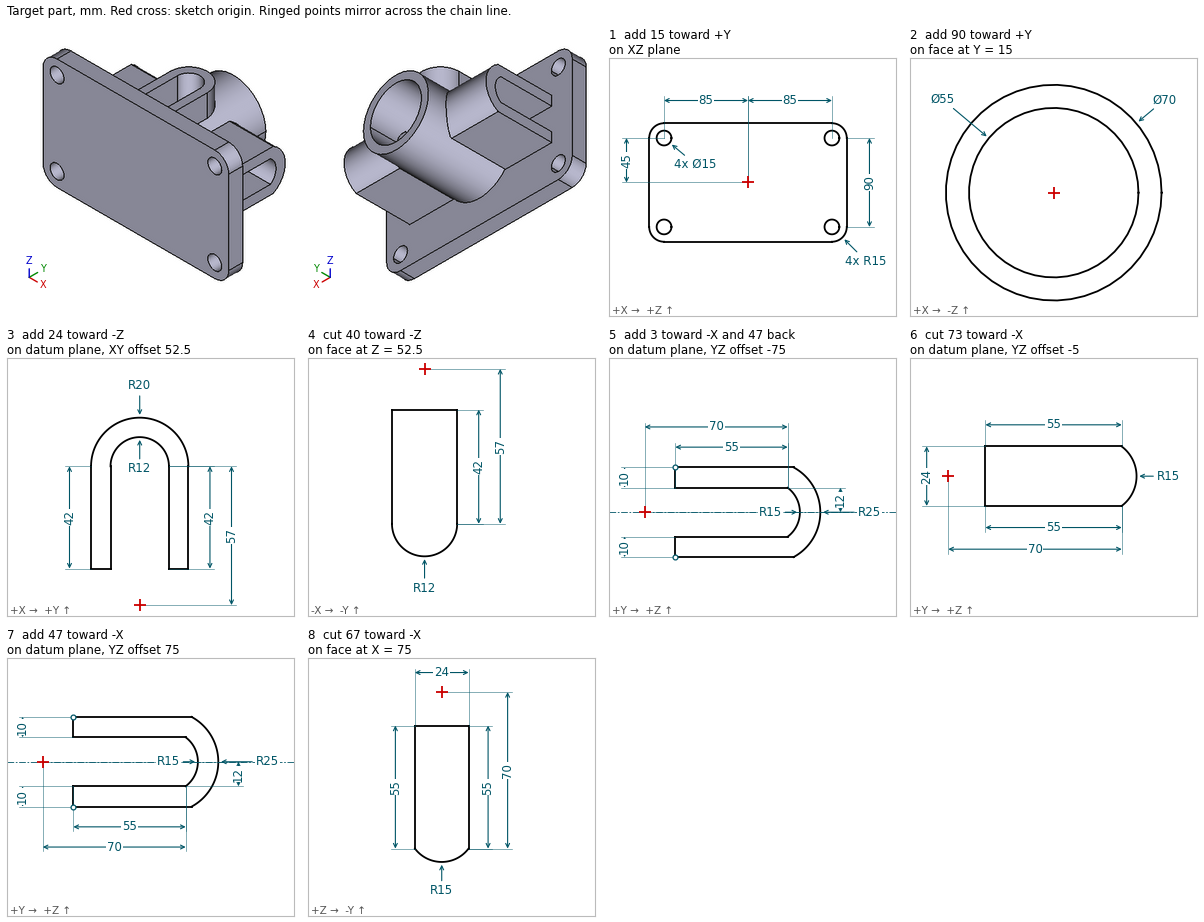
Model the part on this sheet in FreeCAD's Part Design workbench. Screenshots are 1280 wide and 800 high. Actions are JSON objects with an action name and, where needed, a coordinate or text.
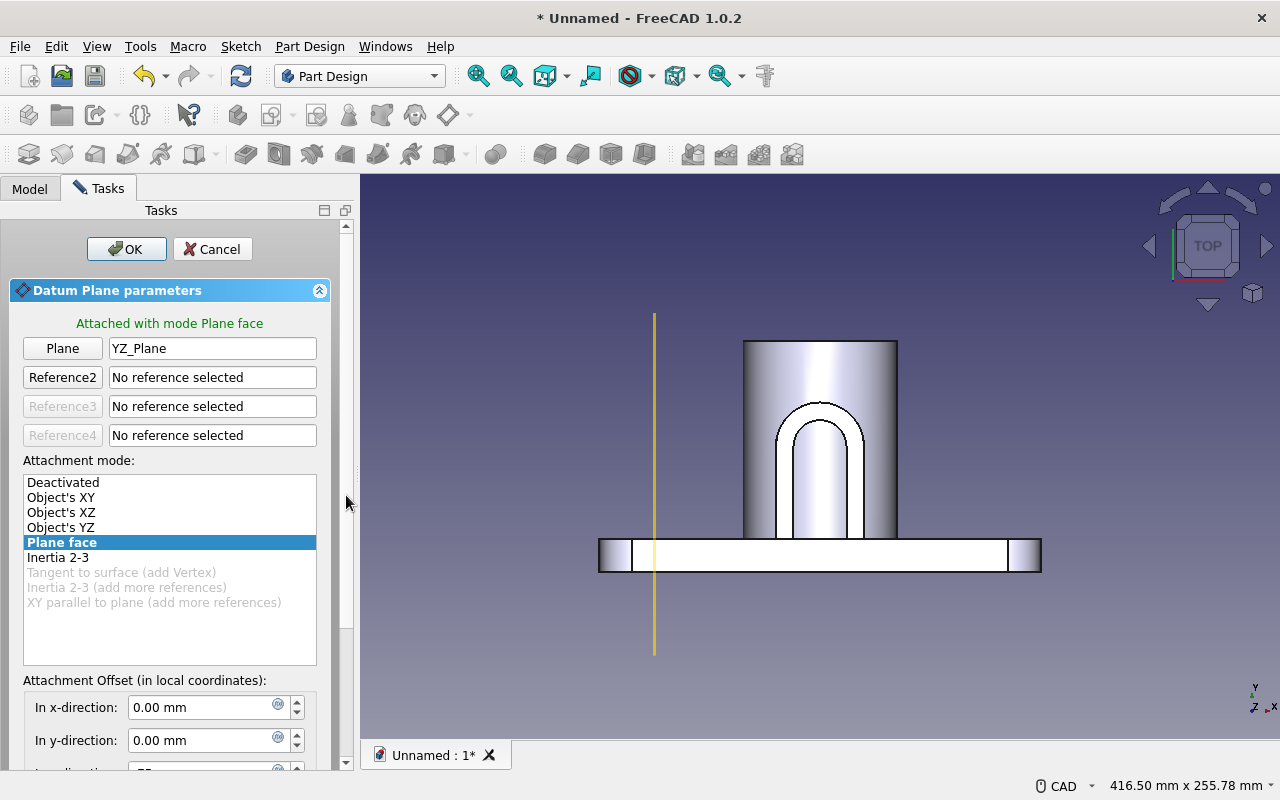
{"action": "left_click", "coordinate": [127, 249]}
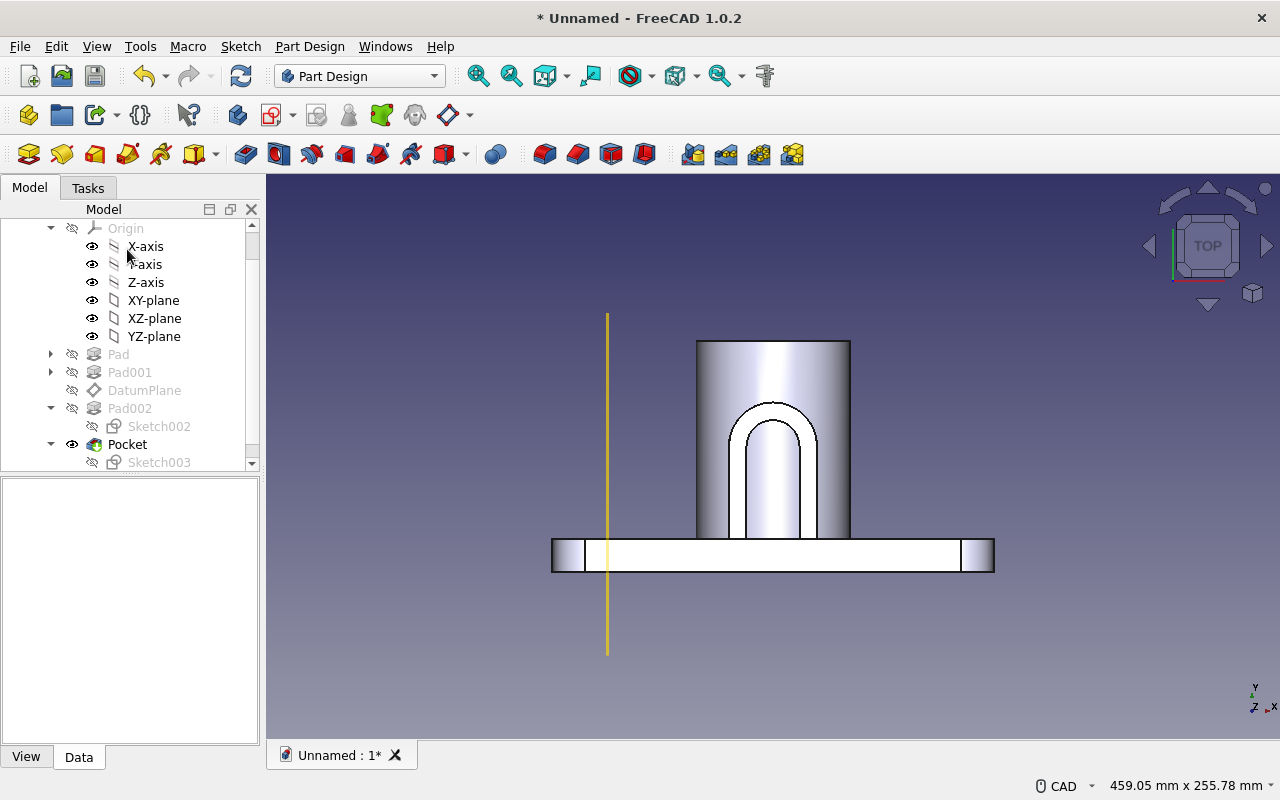
{"action": "scroll", "coordinate": [141, 350], "scroll_direction": "down", "scroll_amount": 3}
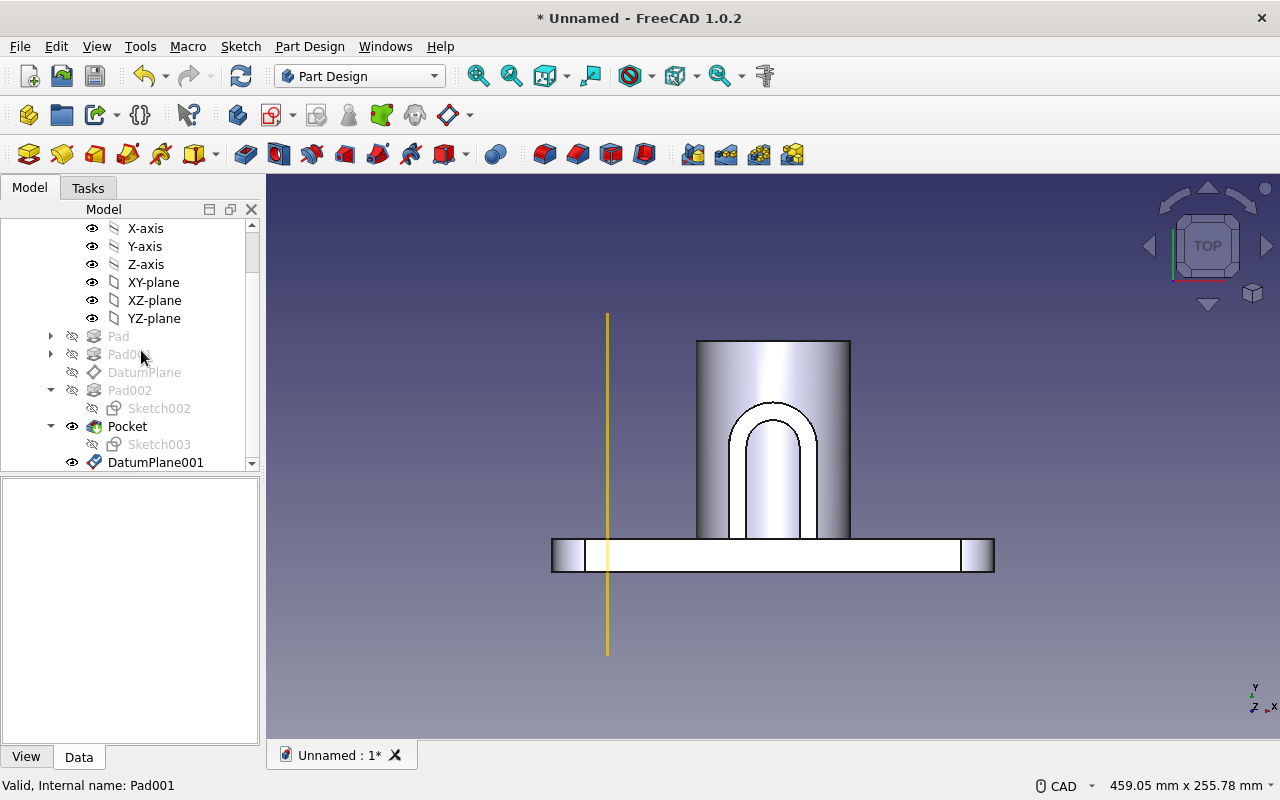
{"action": "left_click", "coordinate": [117, 462]}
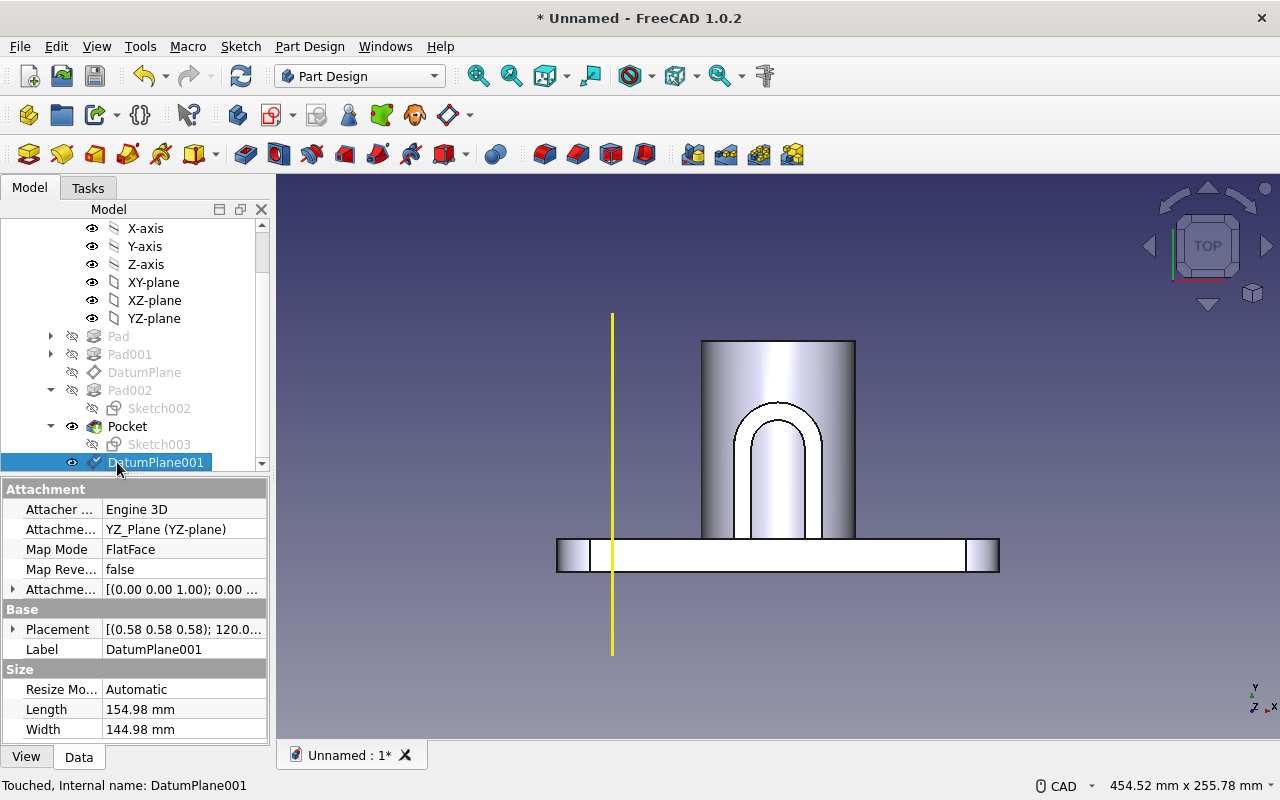
{"action": "left_click", "coordinate": [270, 116]}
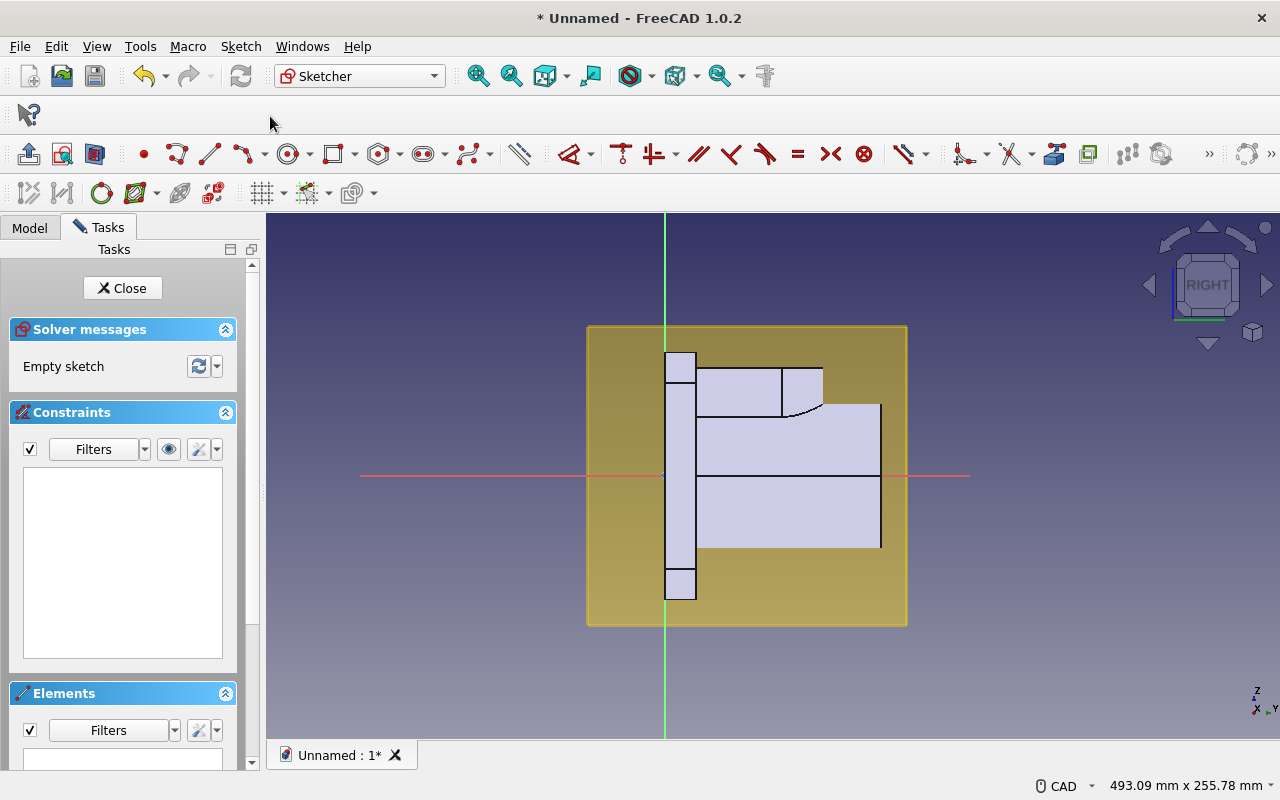
{"action": "key", "text": "q s"}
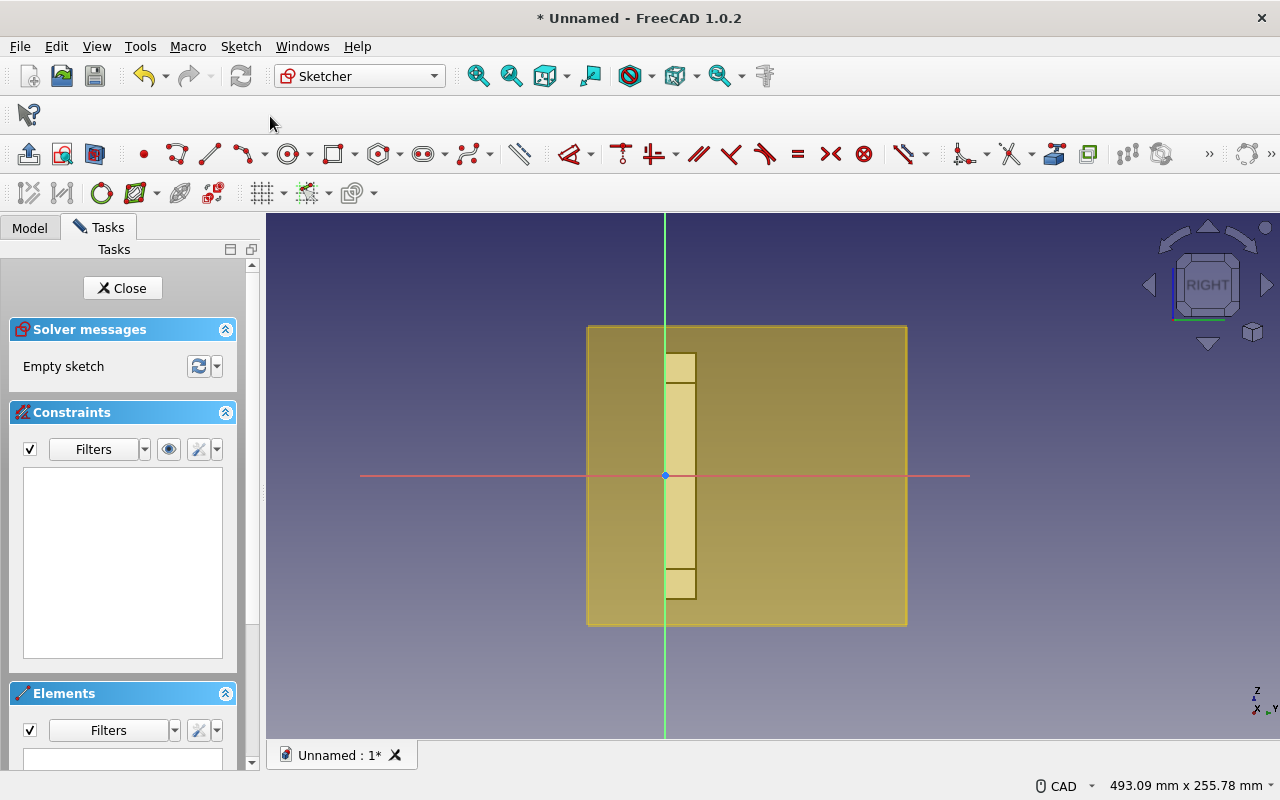
{"action": "scroll", "coordinate": [775, 476], "scroll_direction": "up", "scroll_amount": 6}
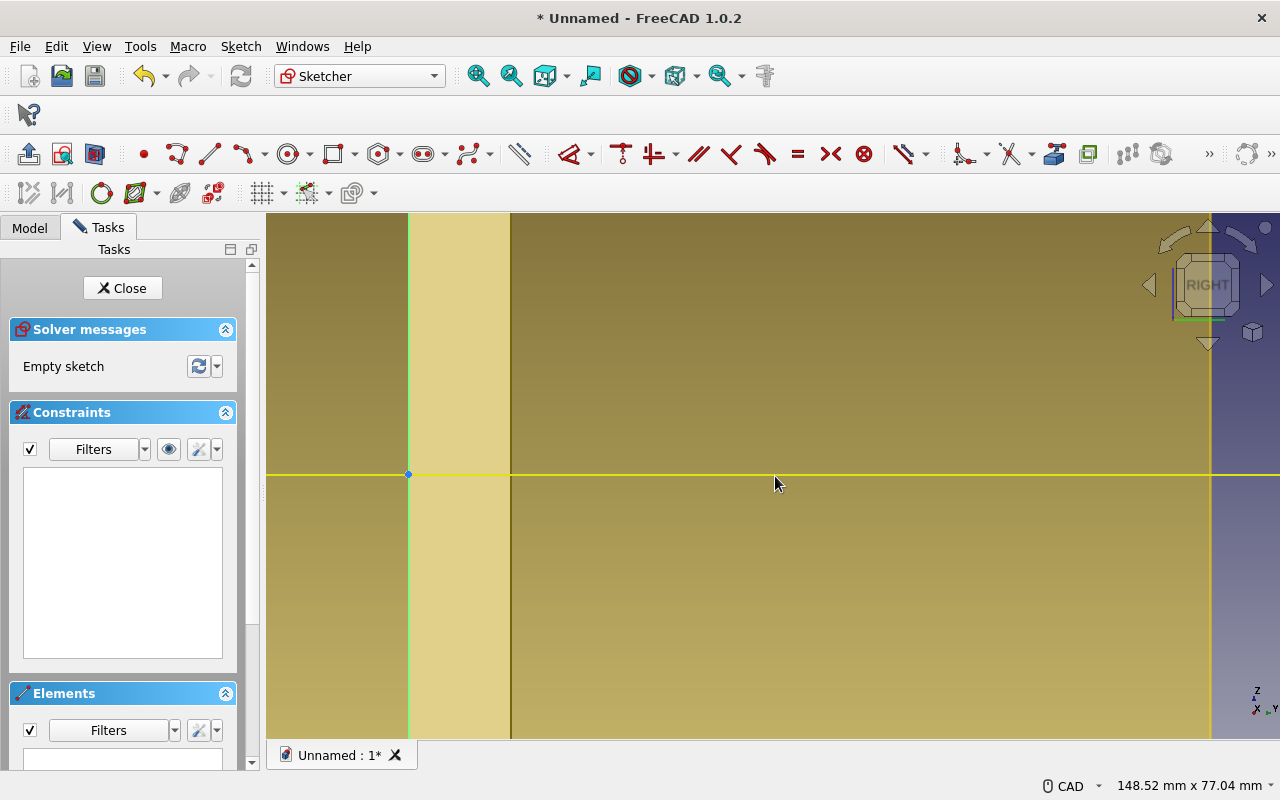
{"action": "left_click", "coordinate": [177, 154]}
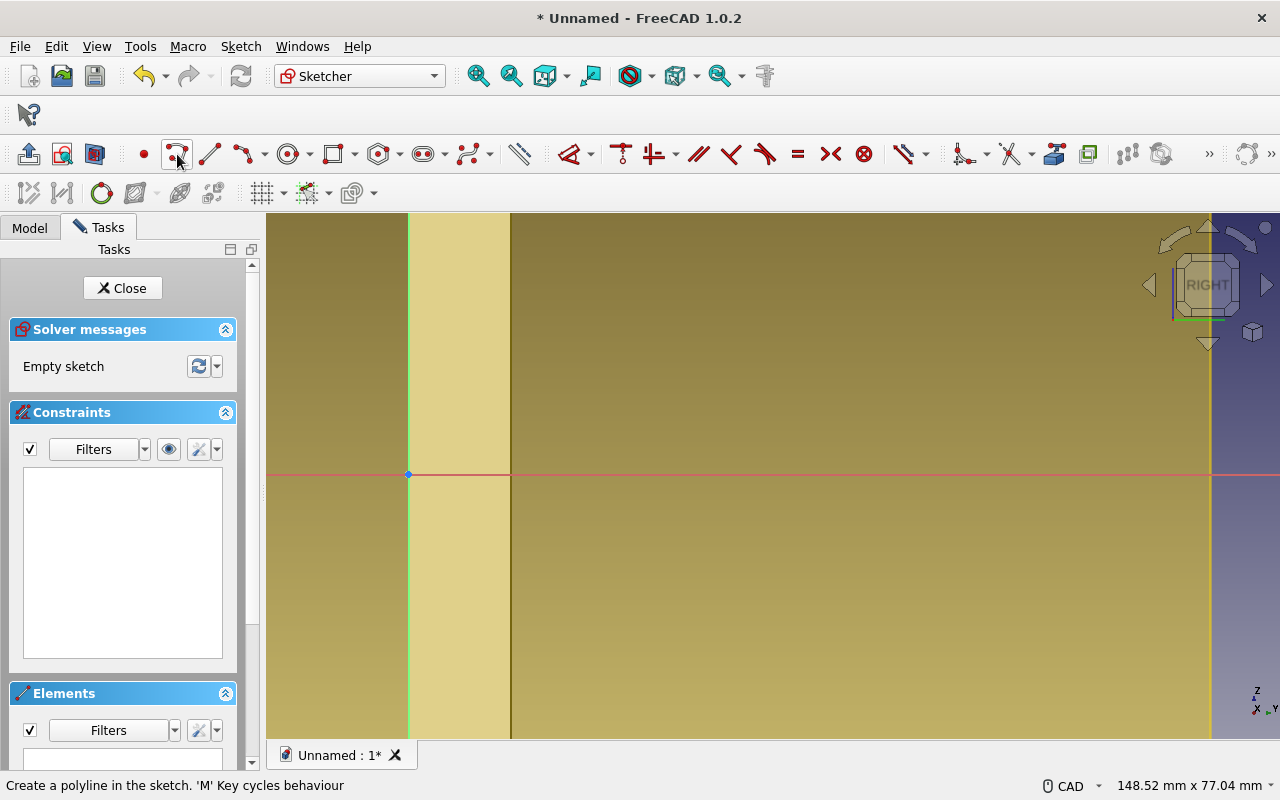
{"action": "left_click", "coordinate": [887, 393]}
{"action": "left_click", "coordinate": [511, 393]}
{"action": "left_click", "coordinate": [511, 325]}
{"action": "left_click", "coordinate": [906, 325]}
{"action": "right_click", "coordinate": [906, 325]}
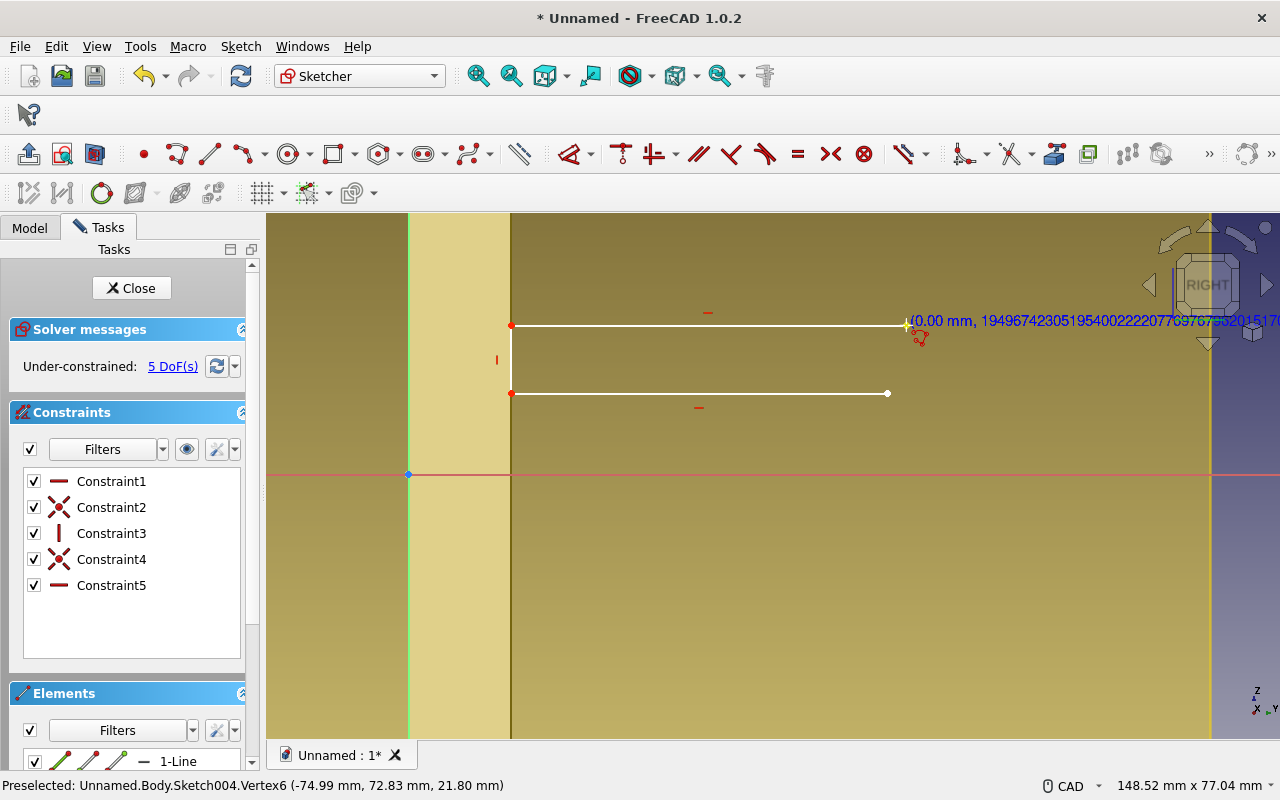
{"action": "left_click", "coordinate": [906, 625]}
{"action": "left_click", "coordinate": [511, 625]}
{"action": "left_click", "coordinate": [511, 557]}
{"action": "left_click", "coordinate": [887, 557]}
{"action": "right_click", "coordinate": [887, 557]}